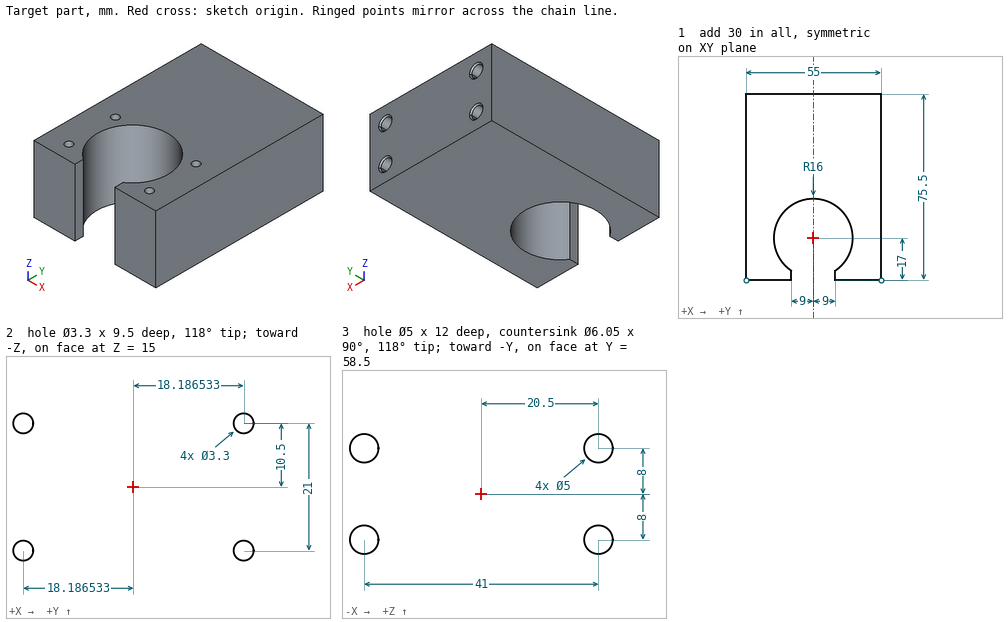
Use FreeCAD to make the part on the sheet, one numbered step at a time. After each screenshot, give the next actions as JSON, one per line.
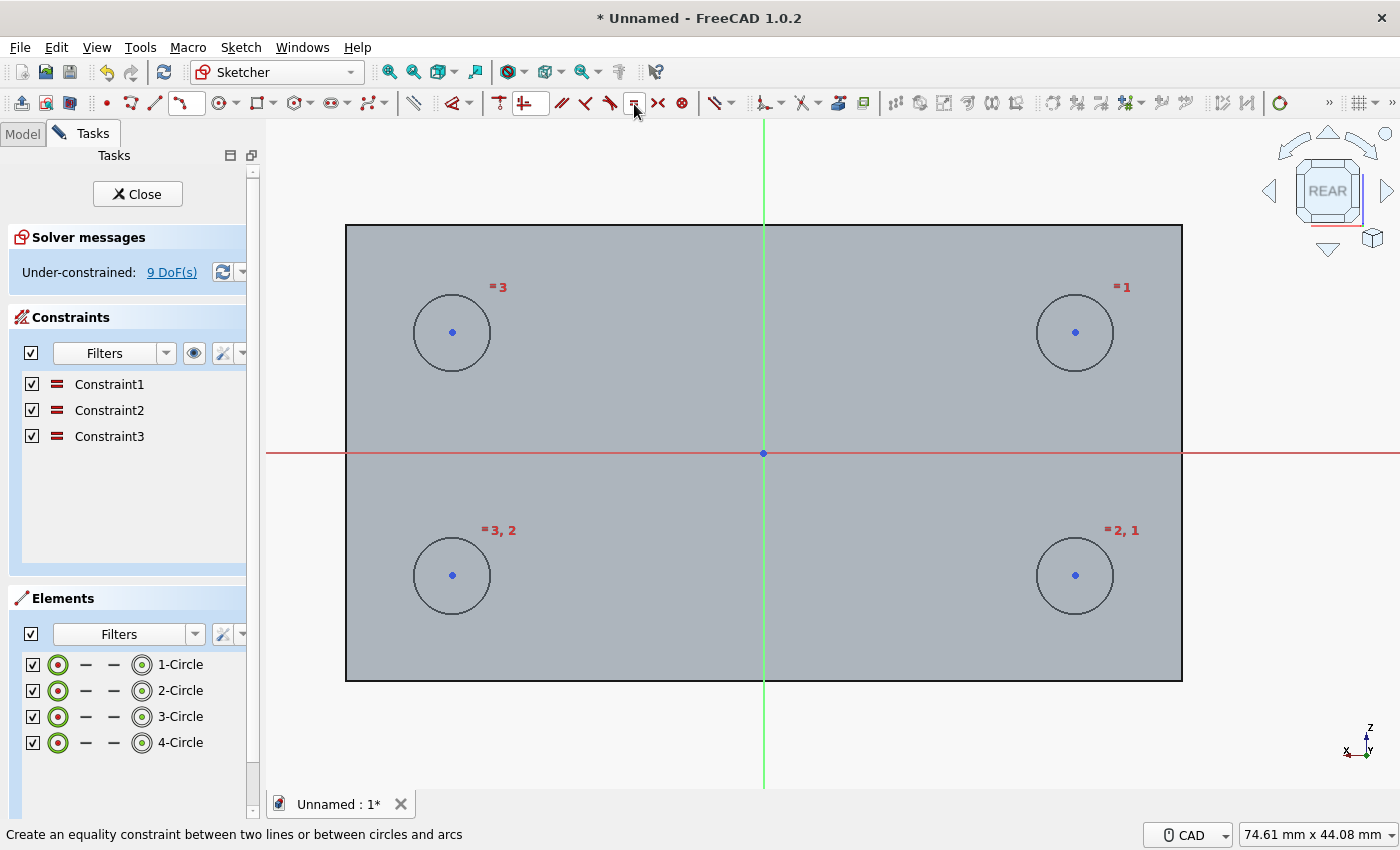
{"action": "left_click", "coordinate": [1075, 333]}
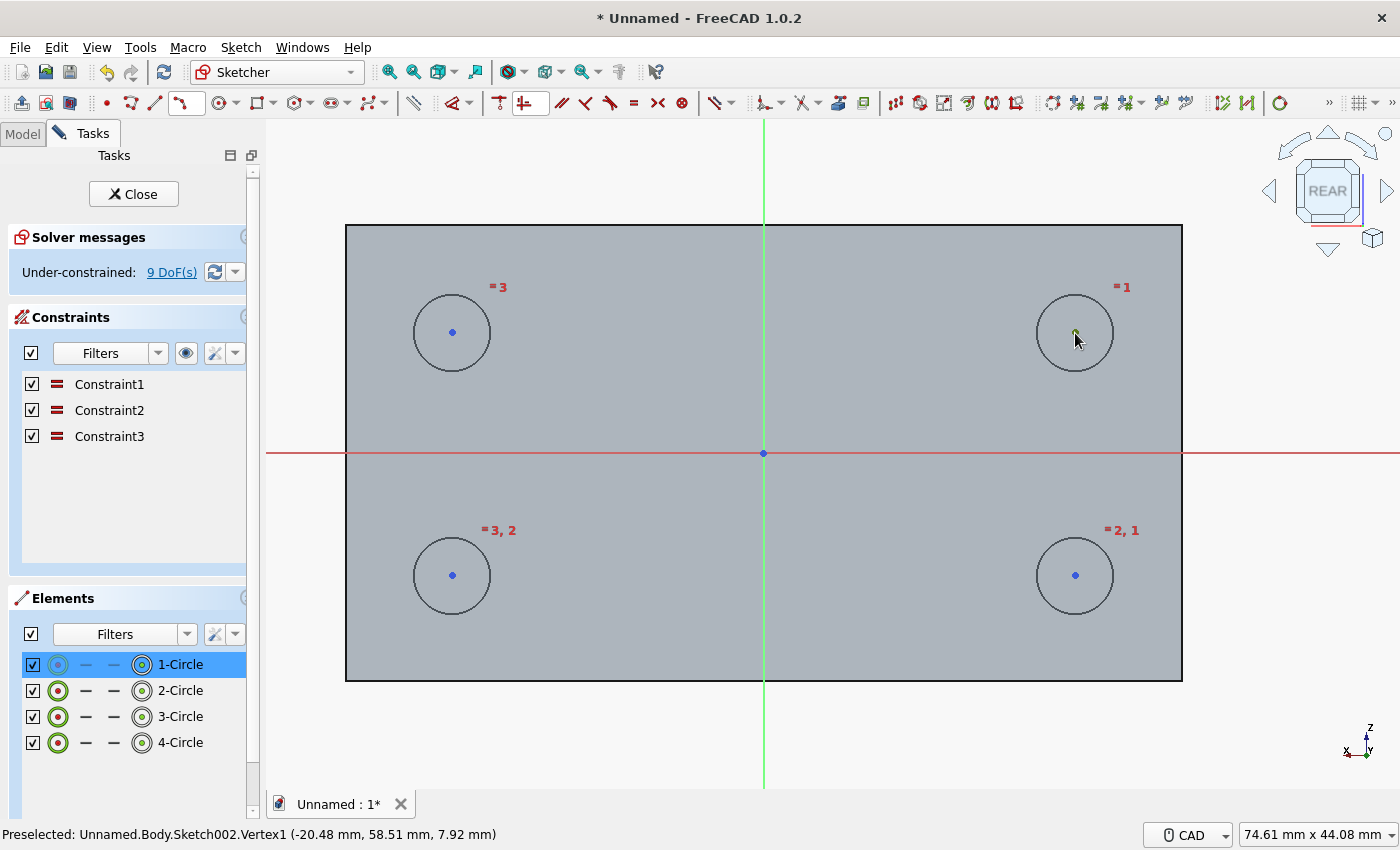
{"action": "left_click", "coordinate": [1075, 576]}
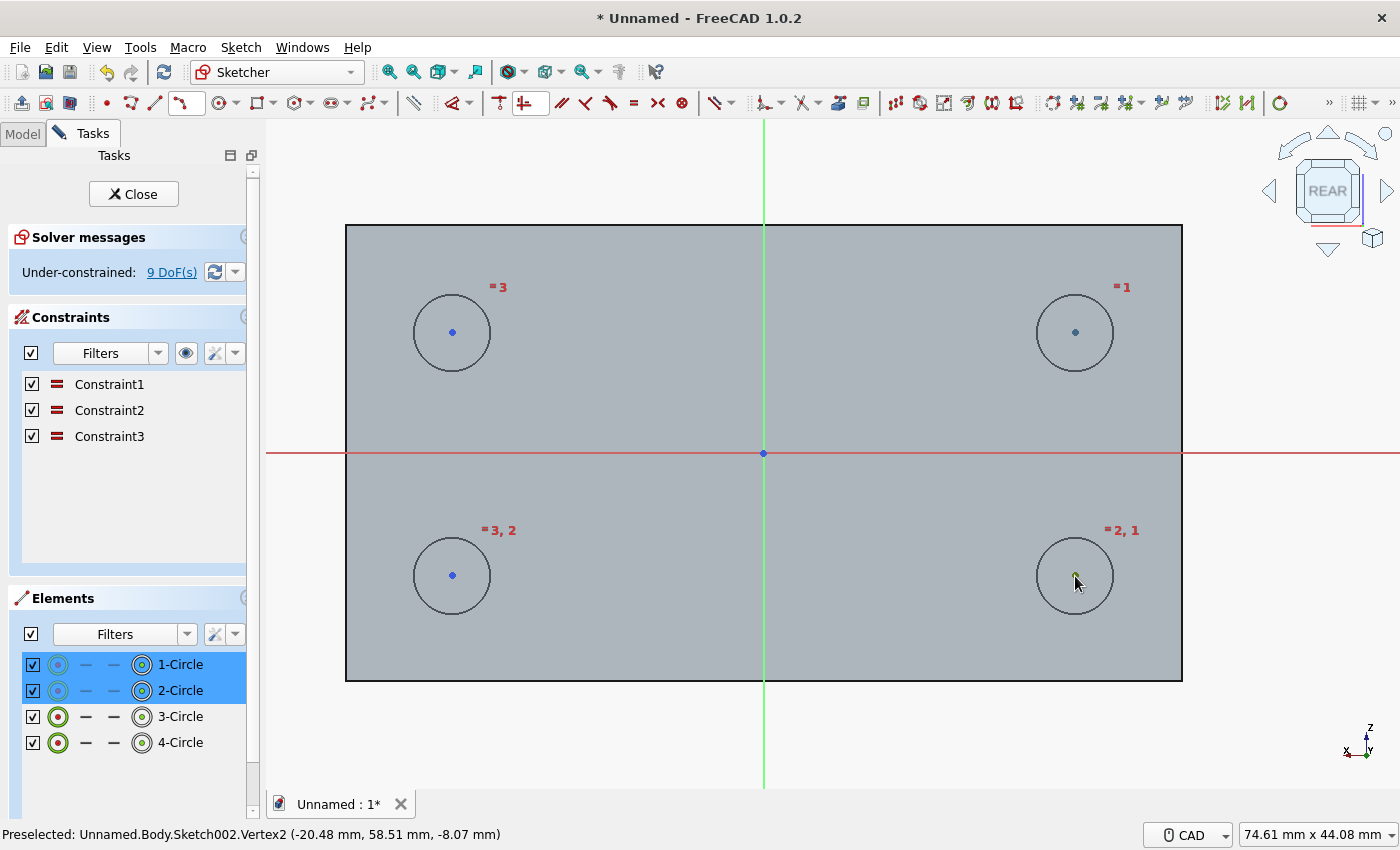
{"action": "key", "text": "v"}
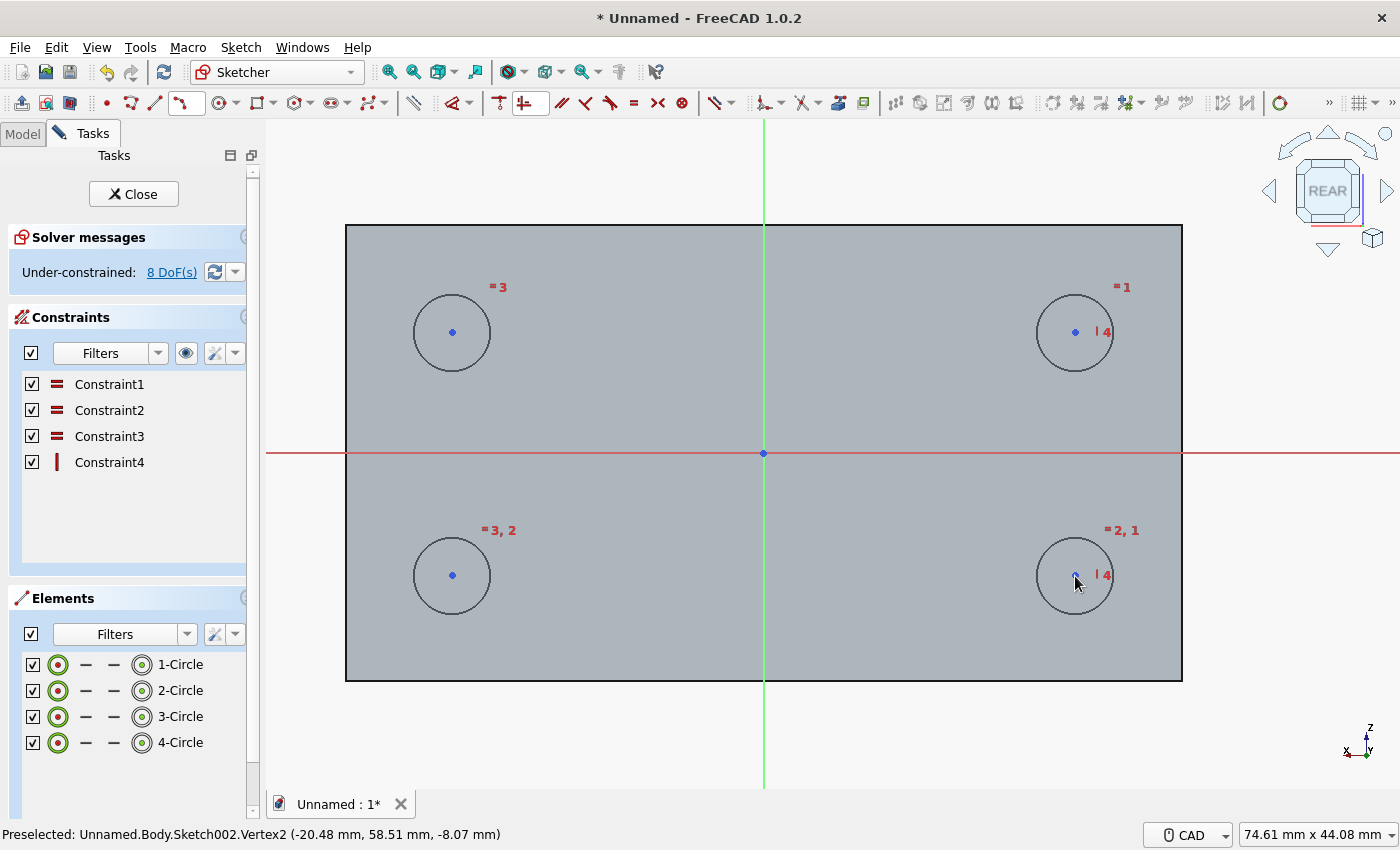
{"action": "left_click", "coordinate": [1075, 576]}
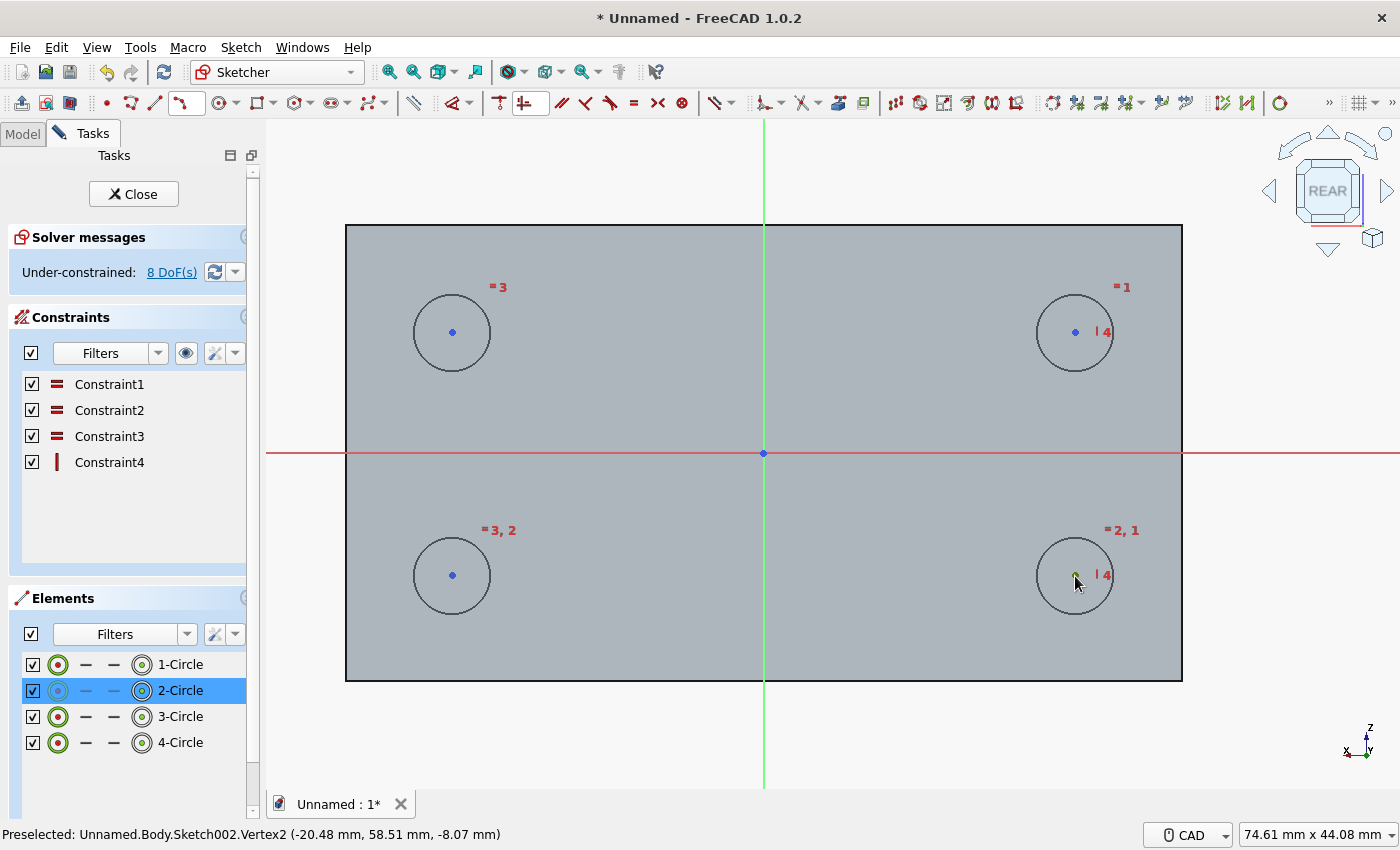
{"action": "left_click", "coordinate": [452, 576]}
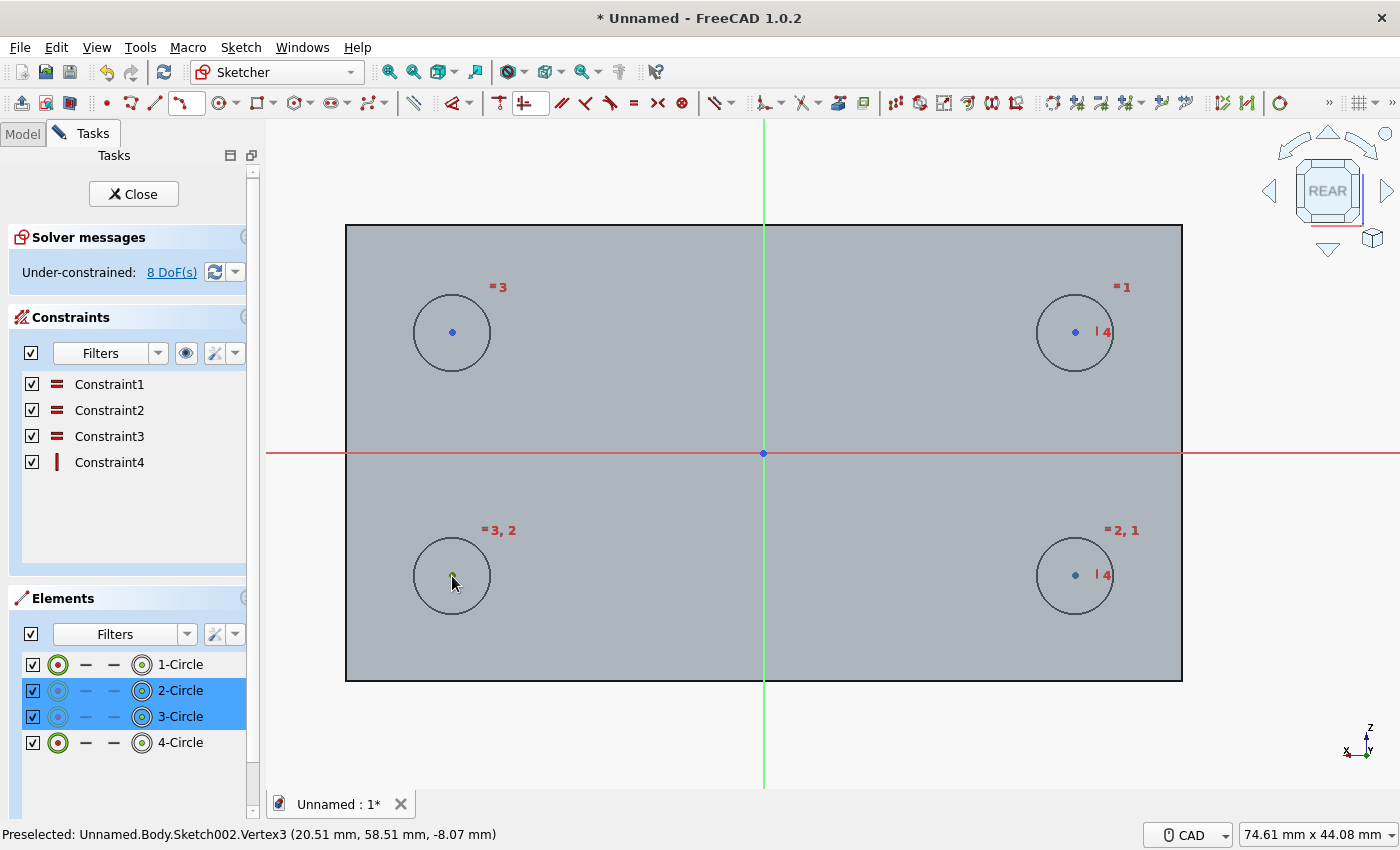
{"action": "left_click", "coordinate": [544, 104]}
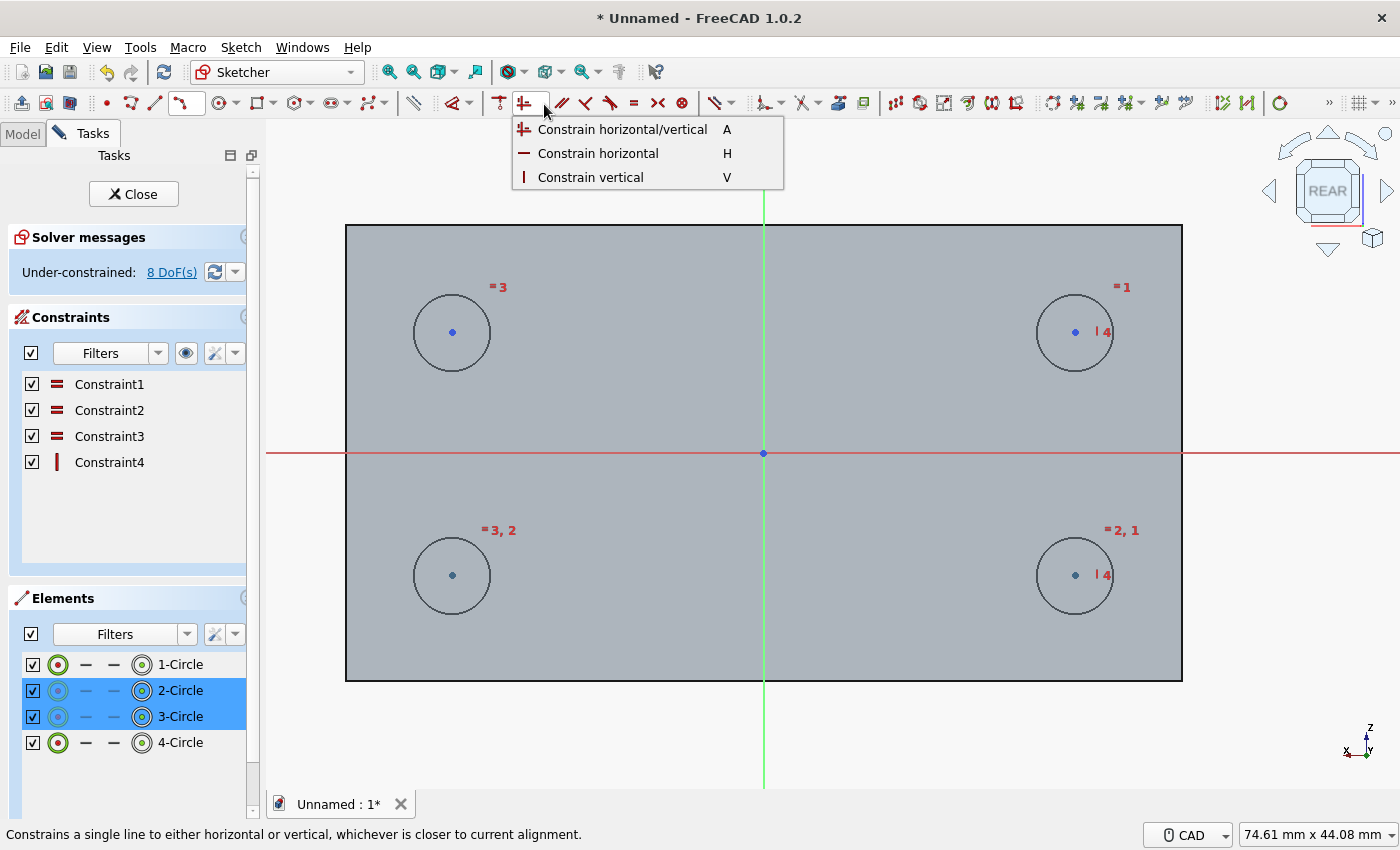
{"action": "left_click", "coordinate": [648, 153]}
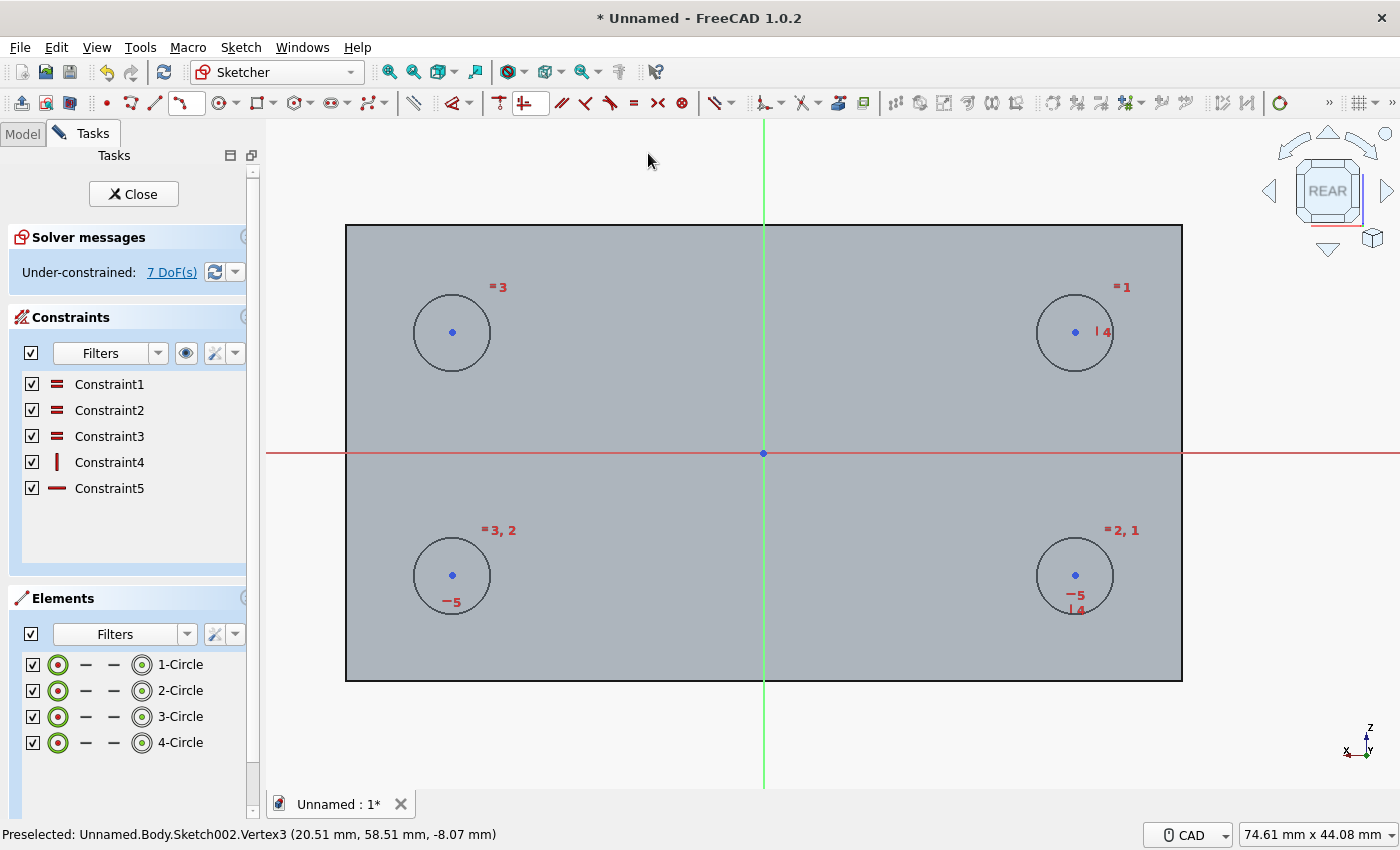
{"action": "left_click", "coordinate": [452, 576]}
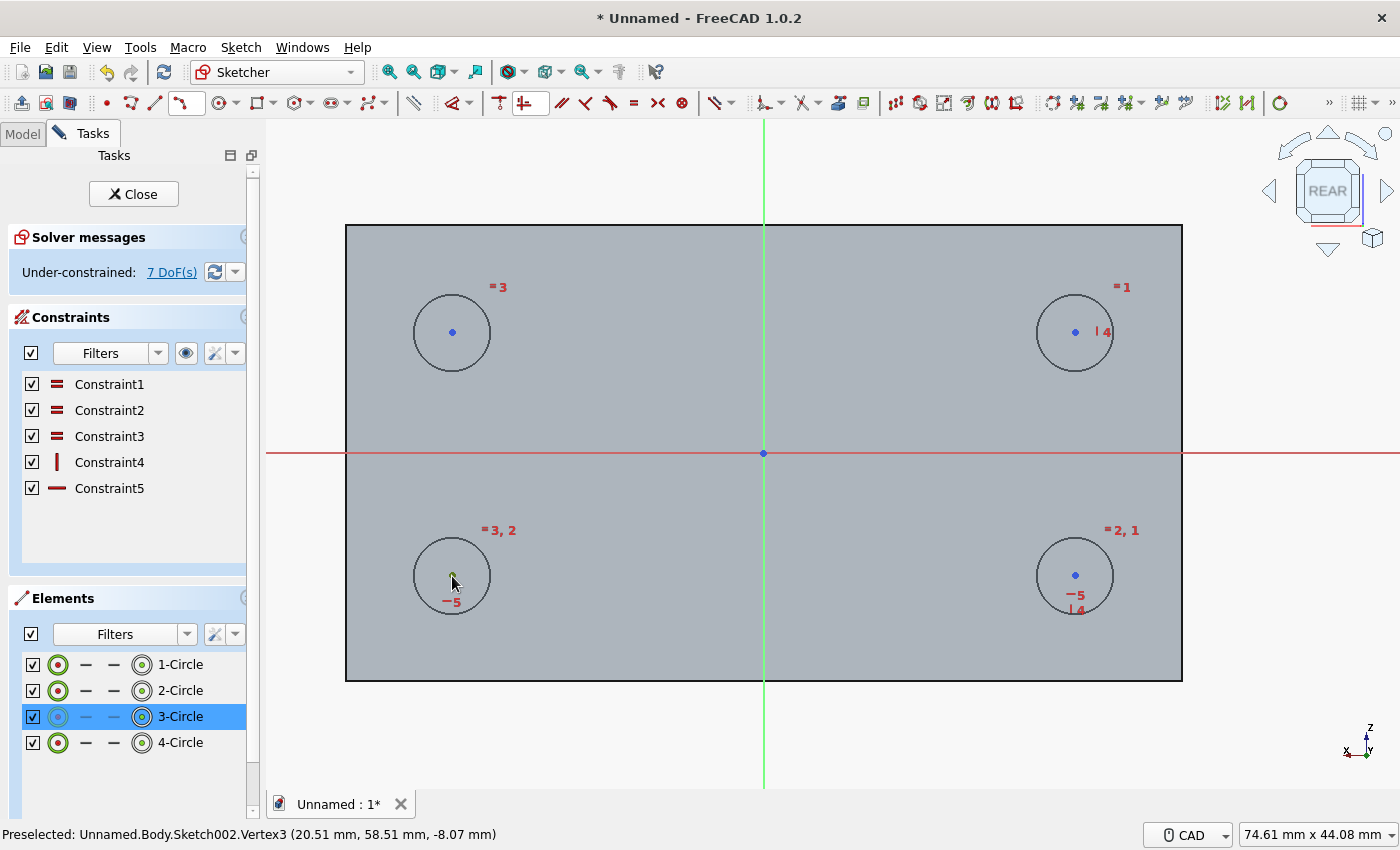
{"action": "left_click", "coordinate": [452, 333]}